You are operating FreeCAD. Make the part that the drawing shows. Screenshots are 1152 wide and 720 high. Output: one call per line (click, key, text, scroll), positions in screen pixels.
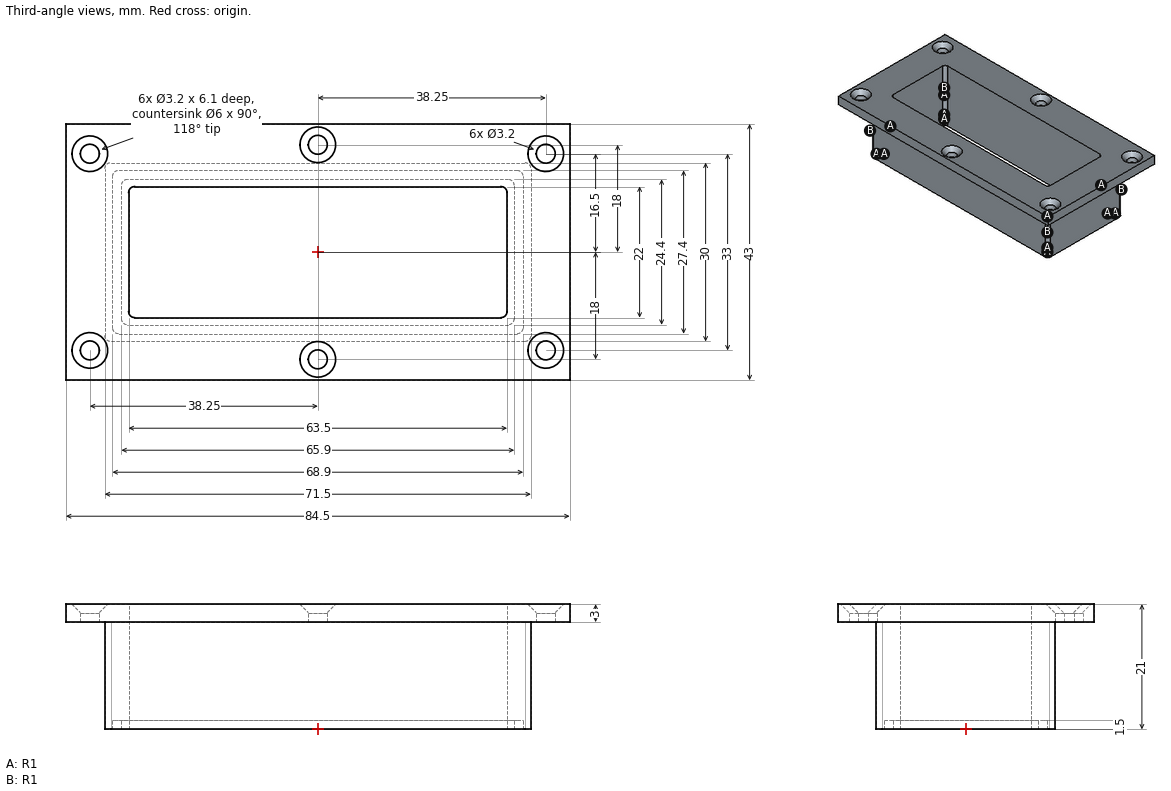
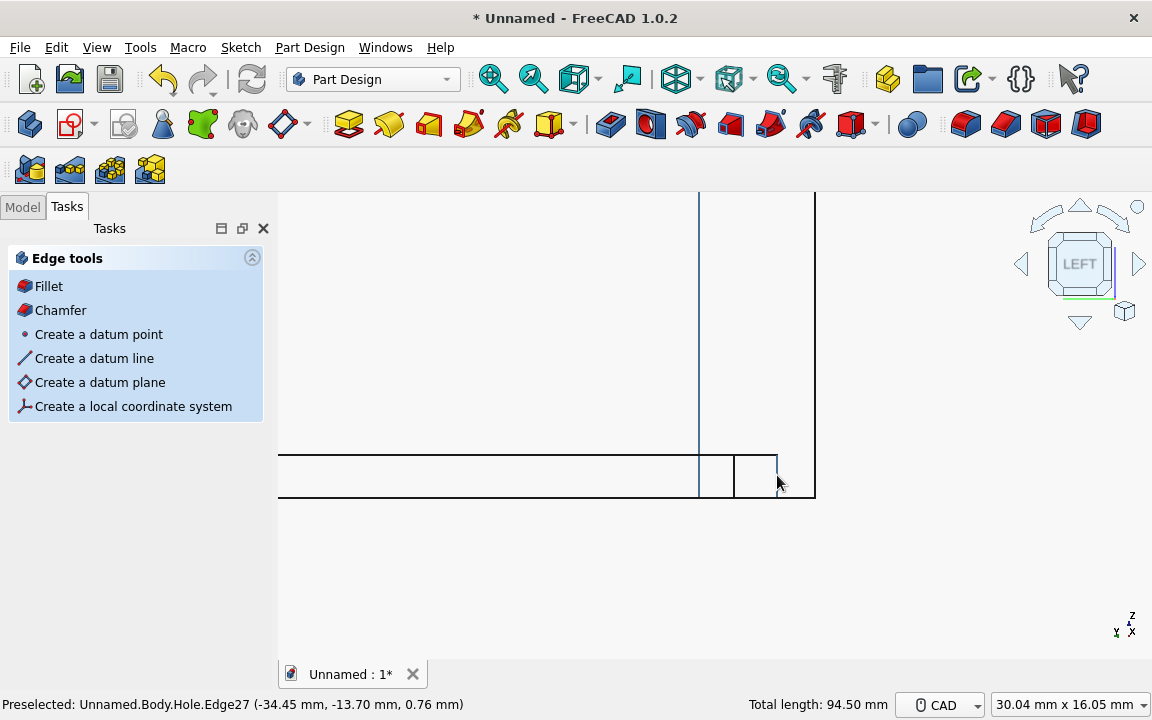
click(734, 475, ctrl)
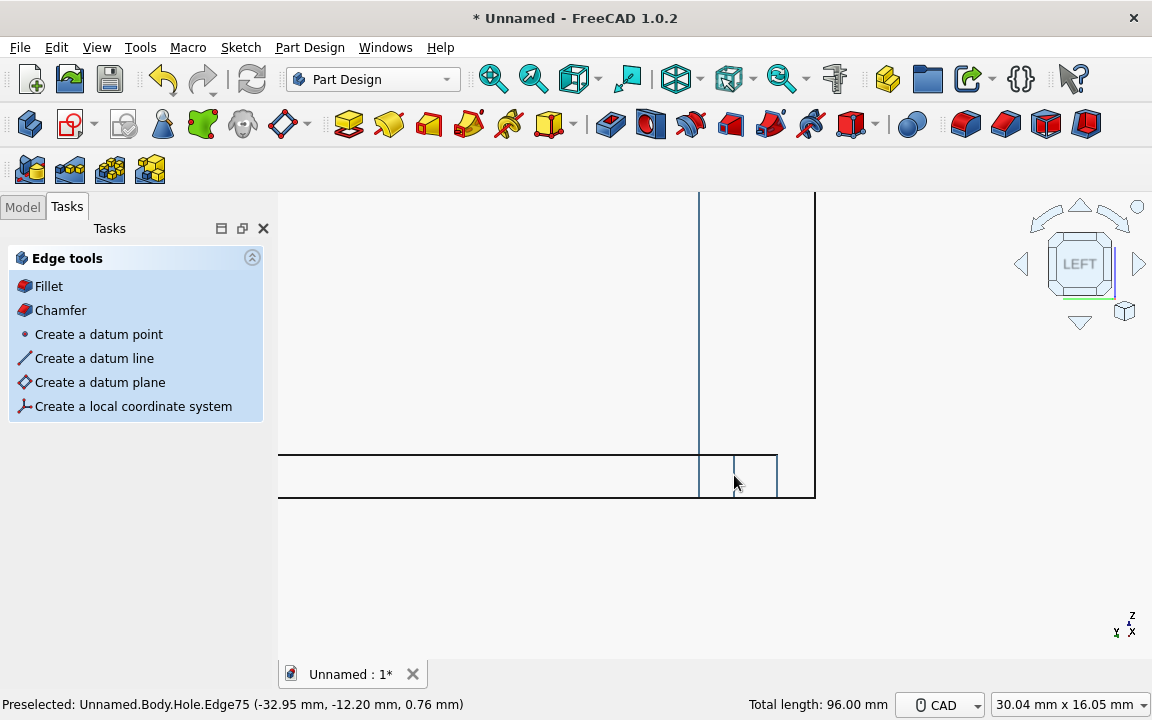
key(v)
key(1)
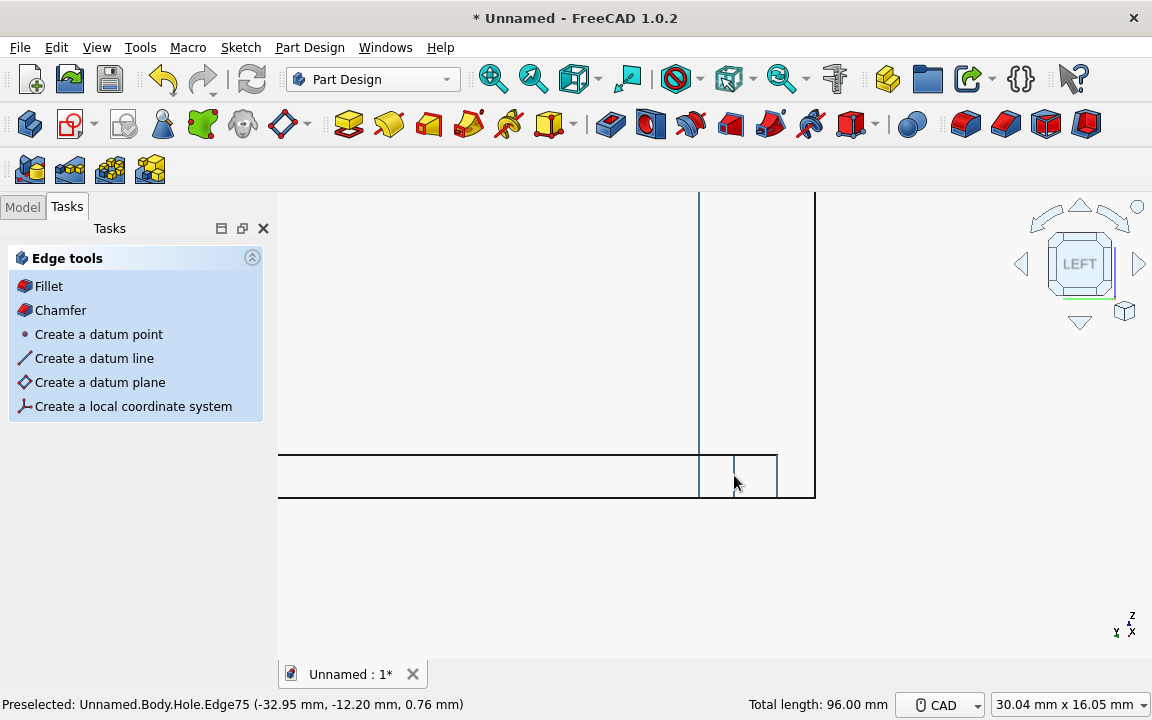
click(966, 124)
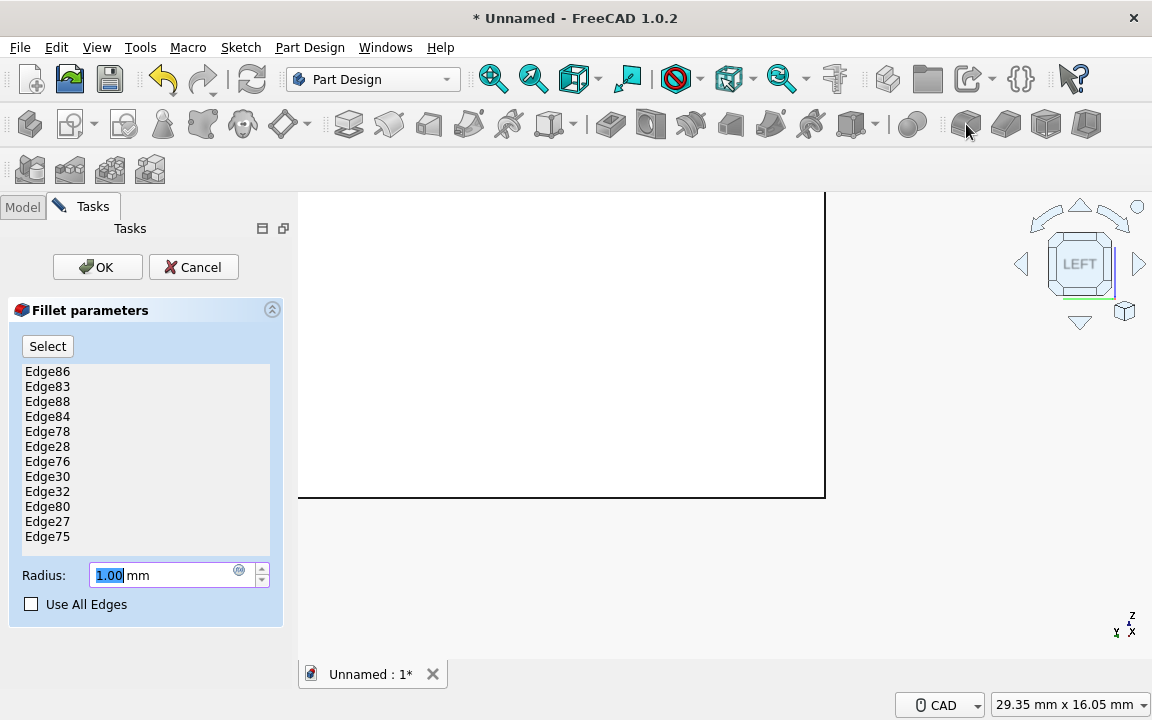
text(1)
key(Tab)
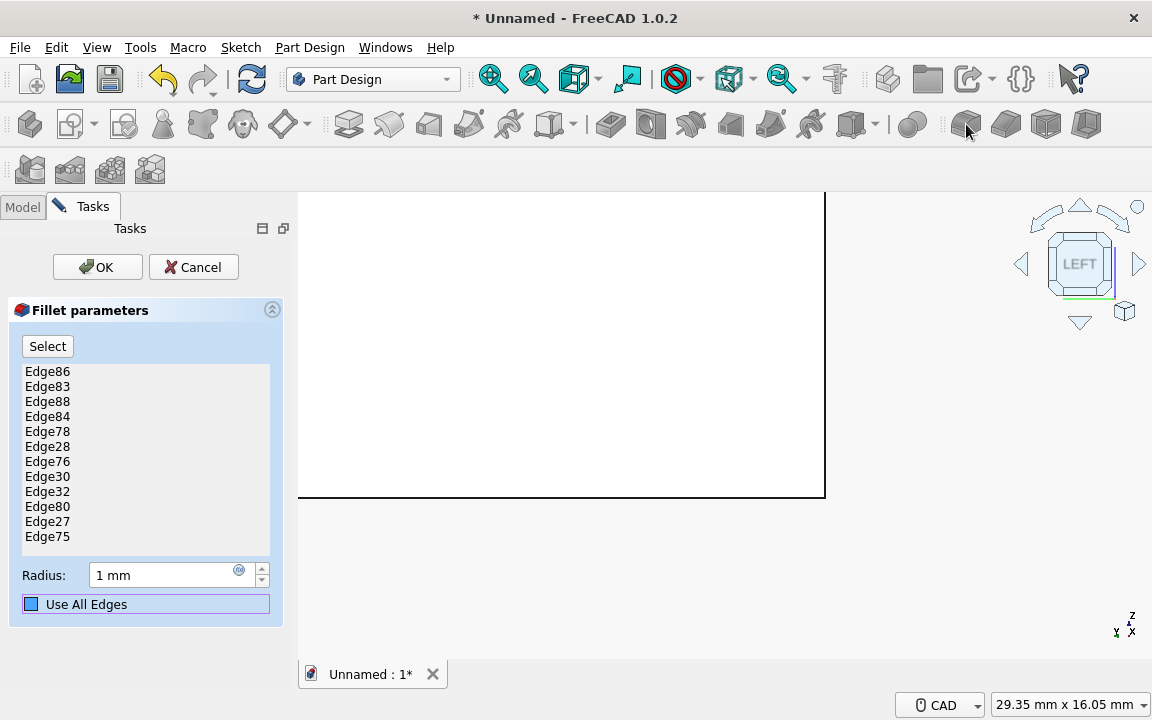
click(98, 267)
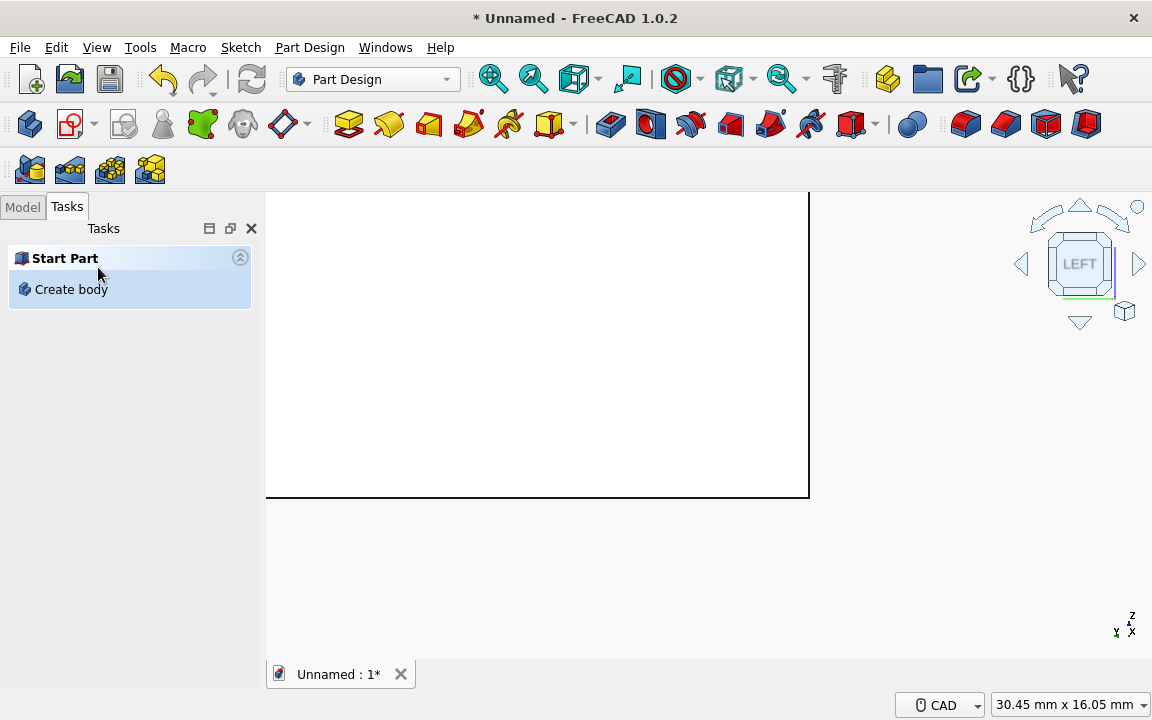
click(494, 80)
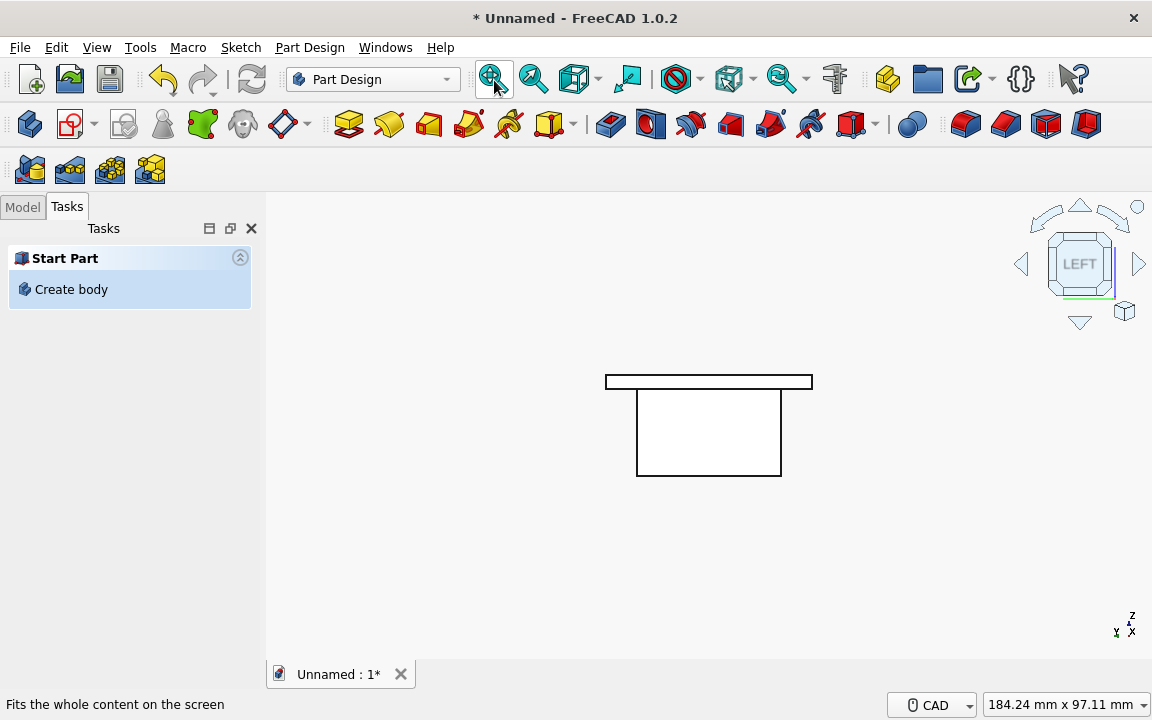
click(781, 432)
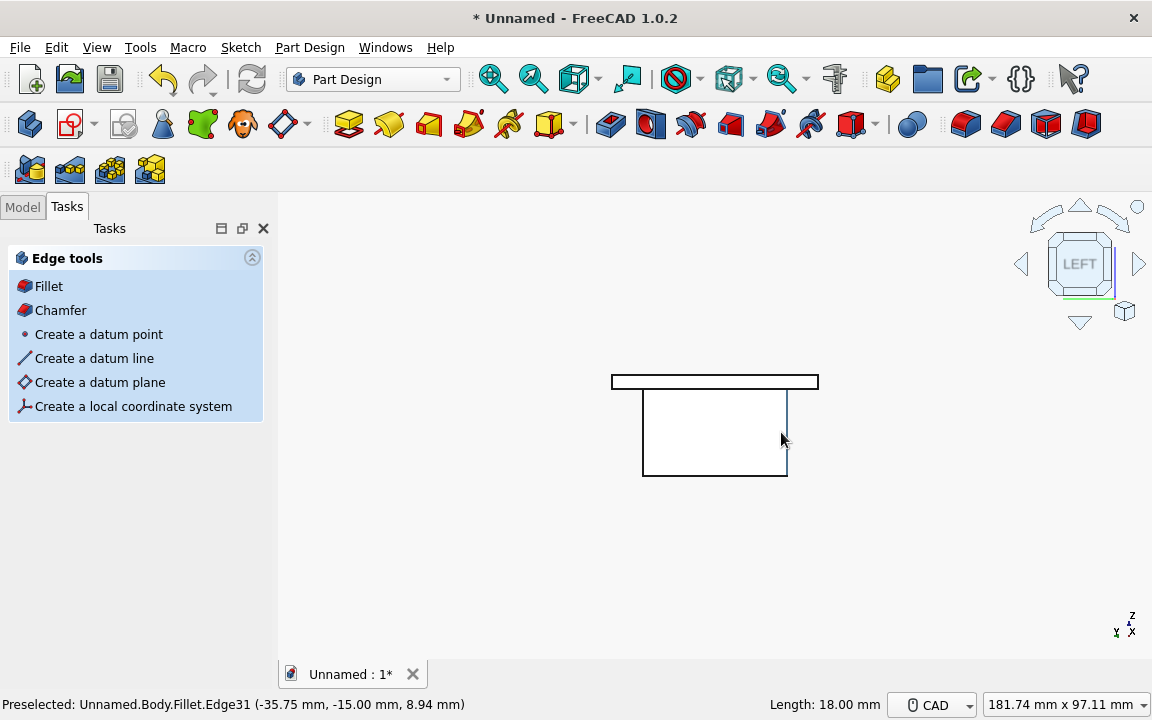
click(643, 432, ctrl)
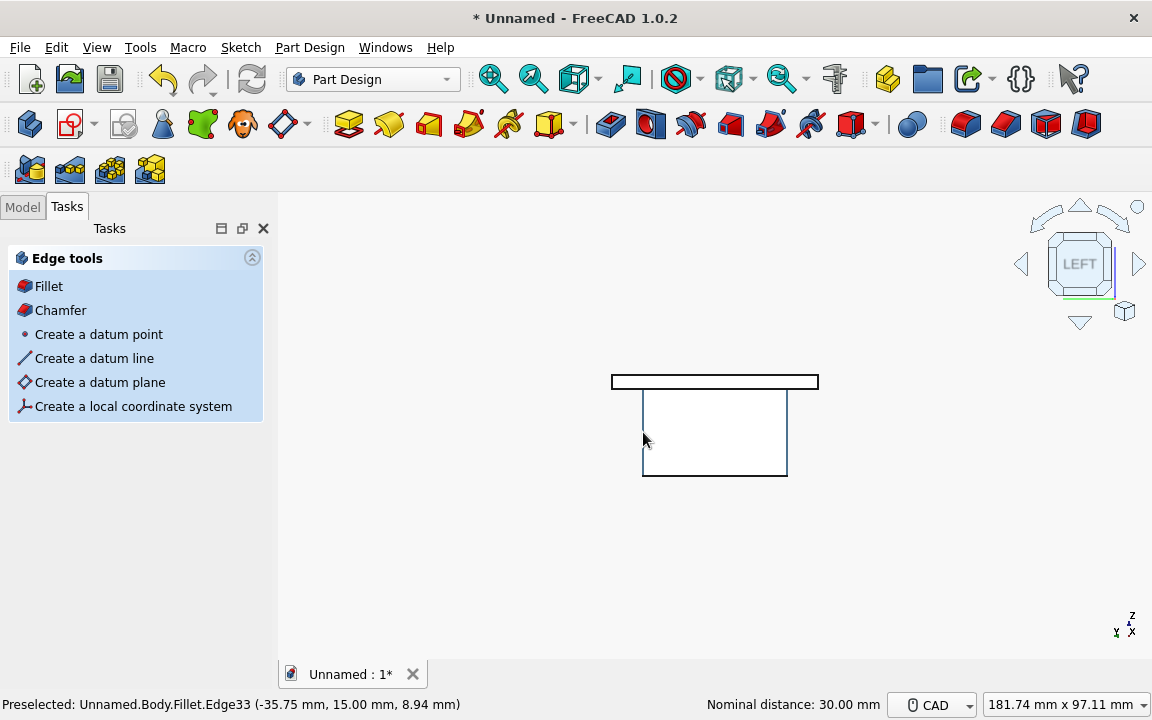
key(0)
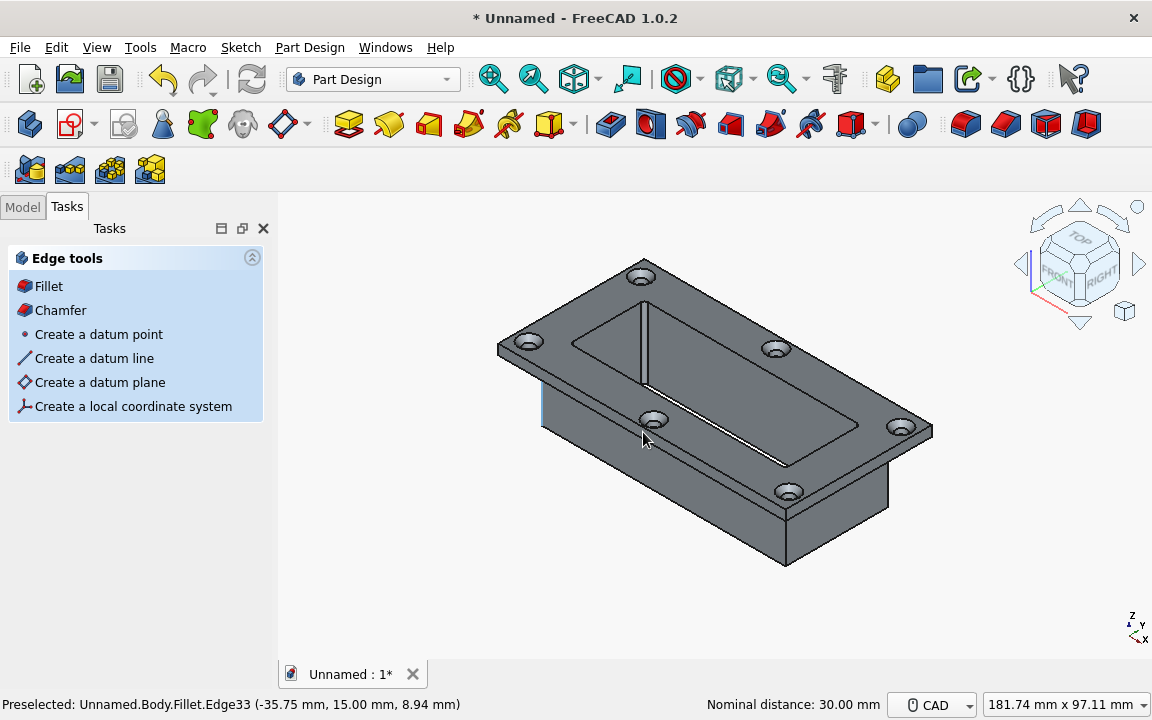
click(786, 530, ctrl)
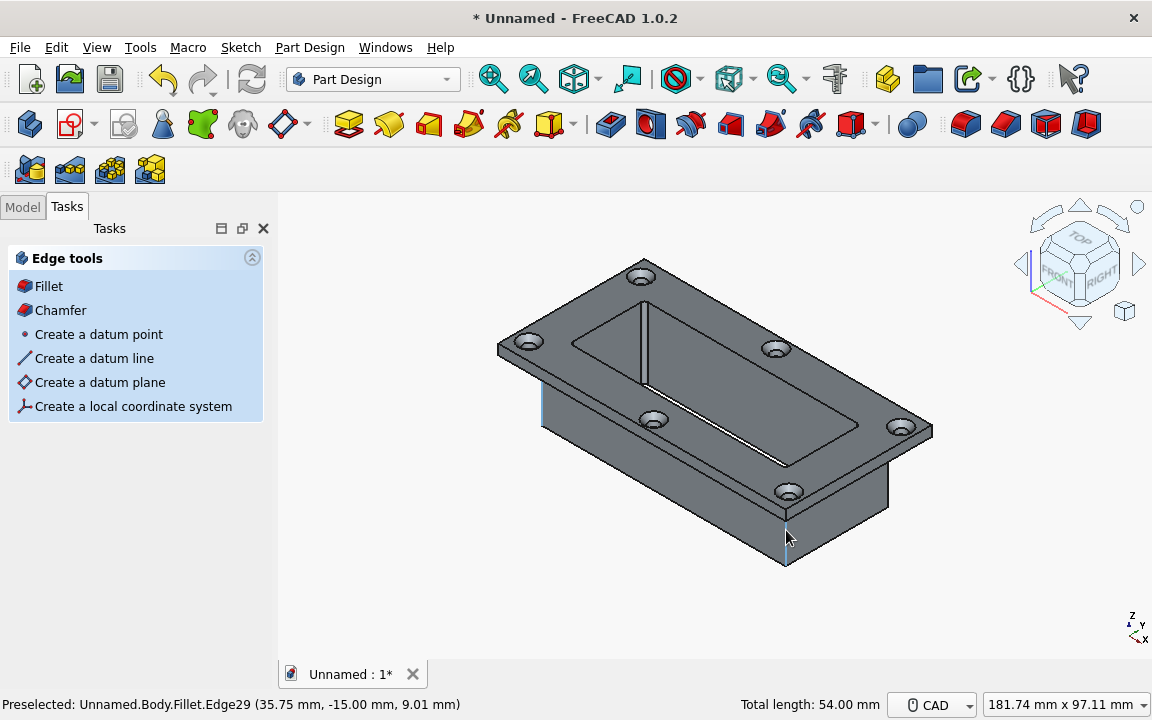
key(2)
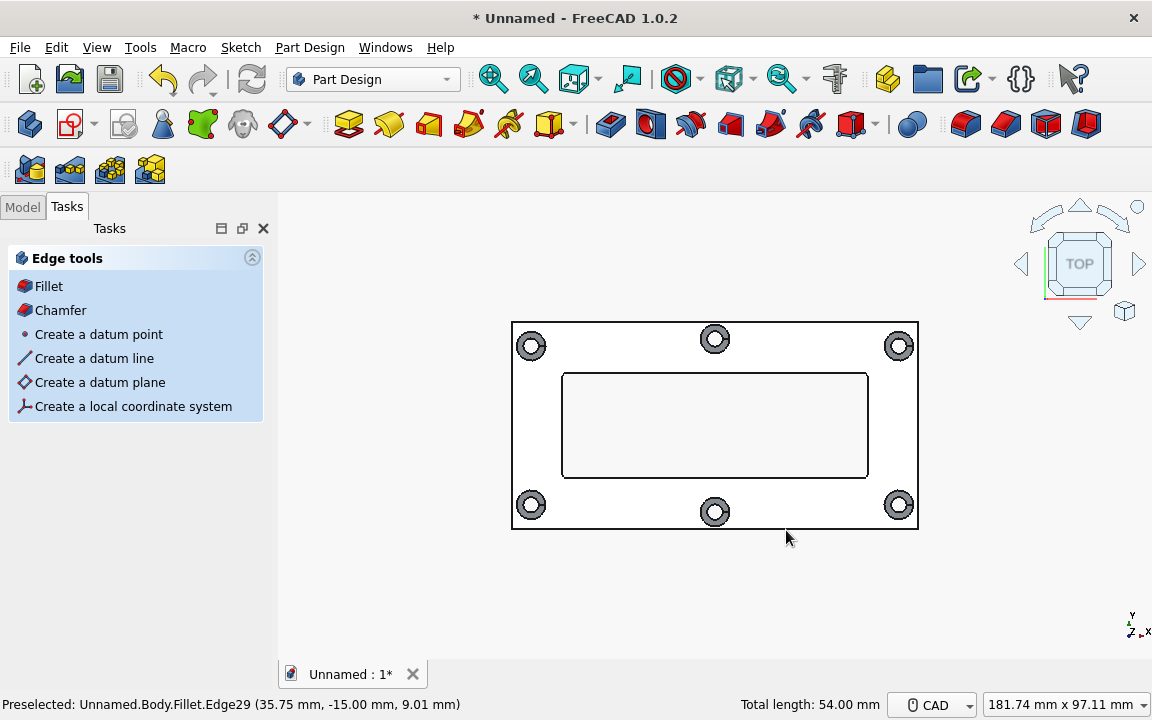
key(1)